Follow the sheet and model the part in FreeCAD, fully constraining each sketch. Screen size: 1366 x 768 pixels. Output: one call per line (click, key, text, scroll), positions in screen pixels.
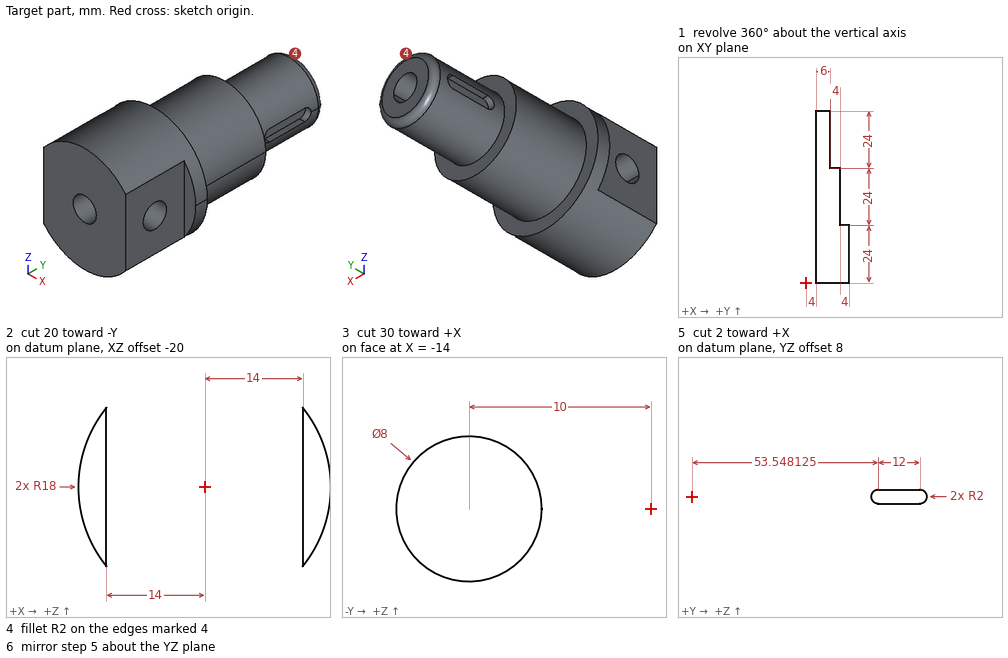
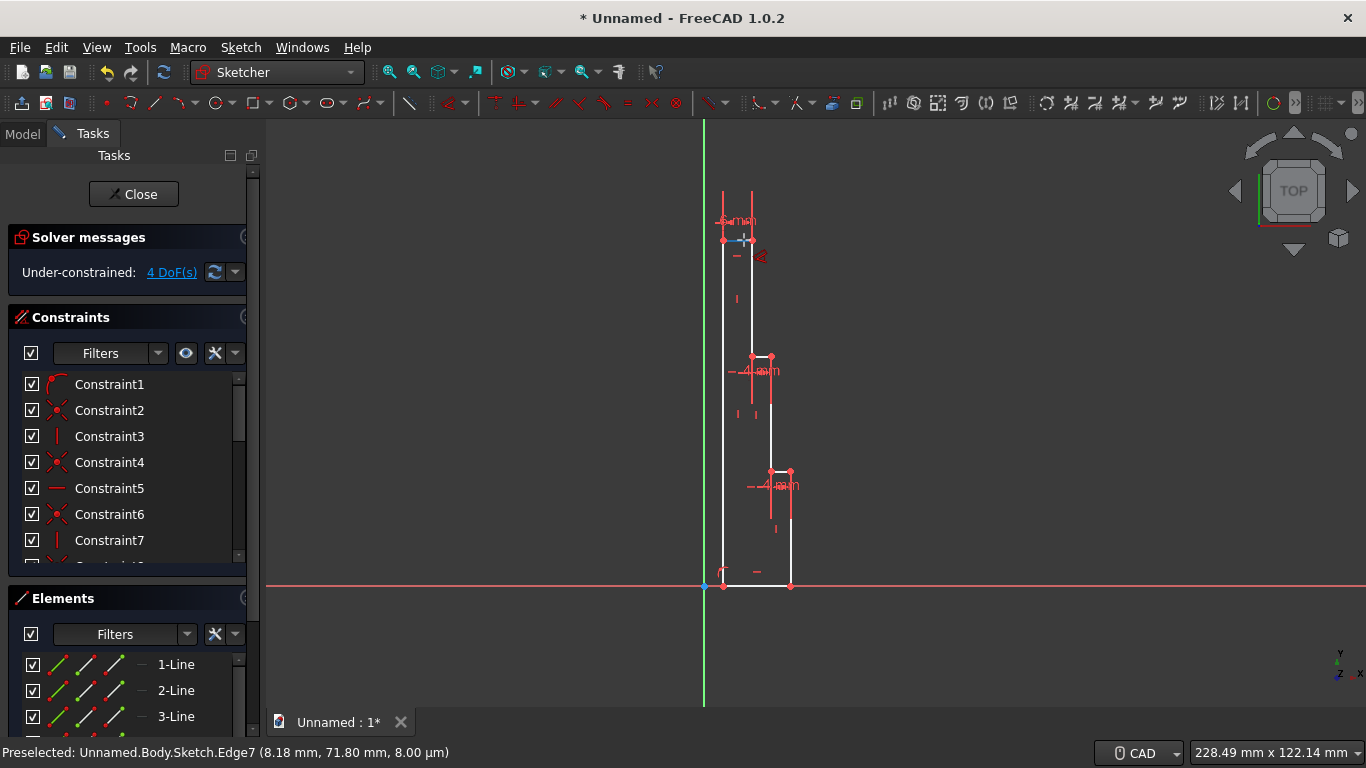
click(791, 552)
click(825, 529)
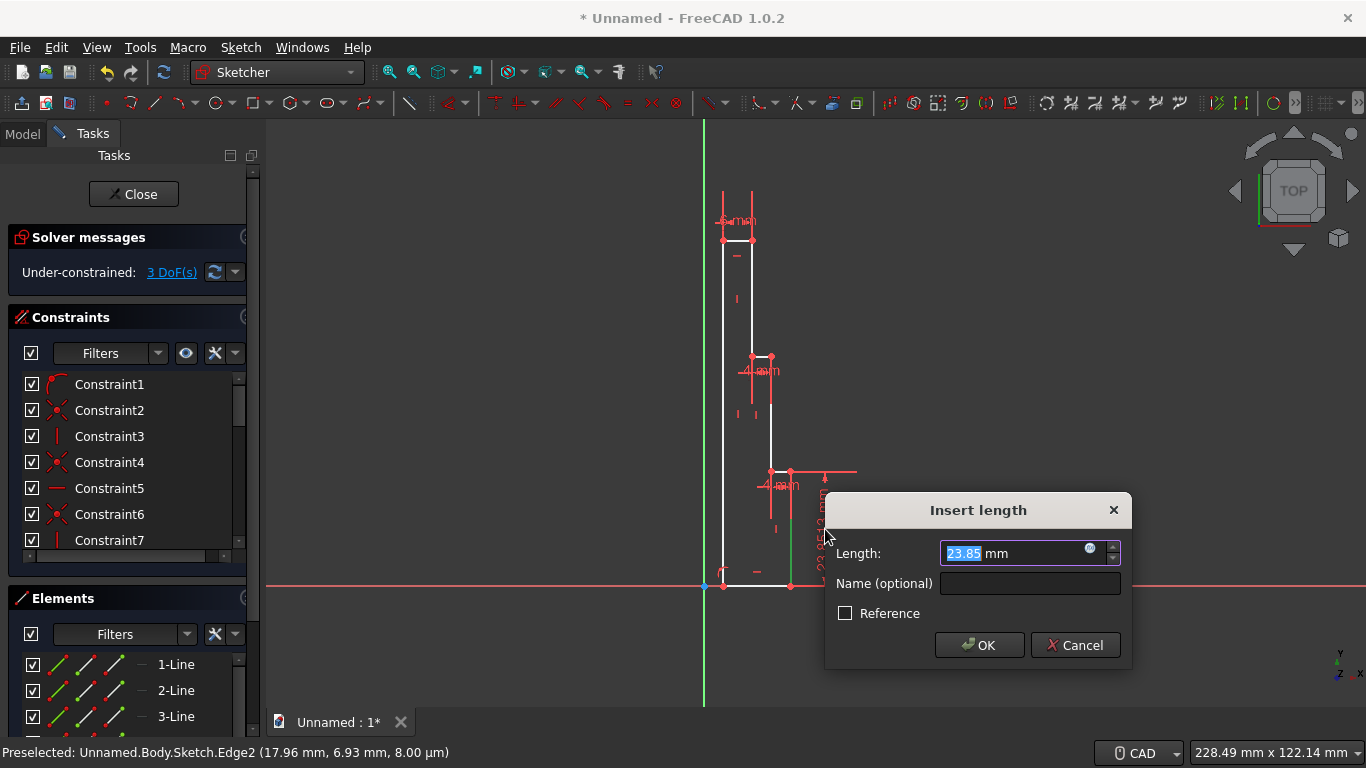
text(24)
key(Return)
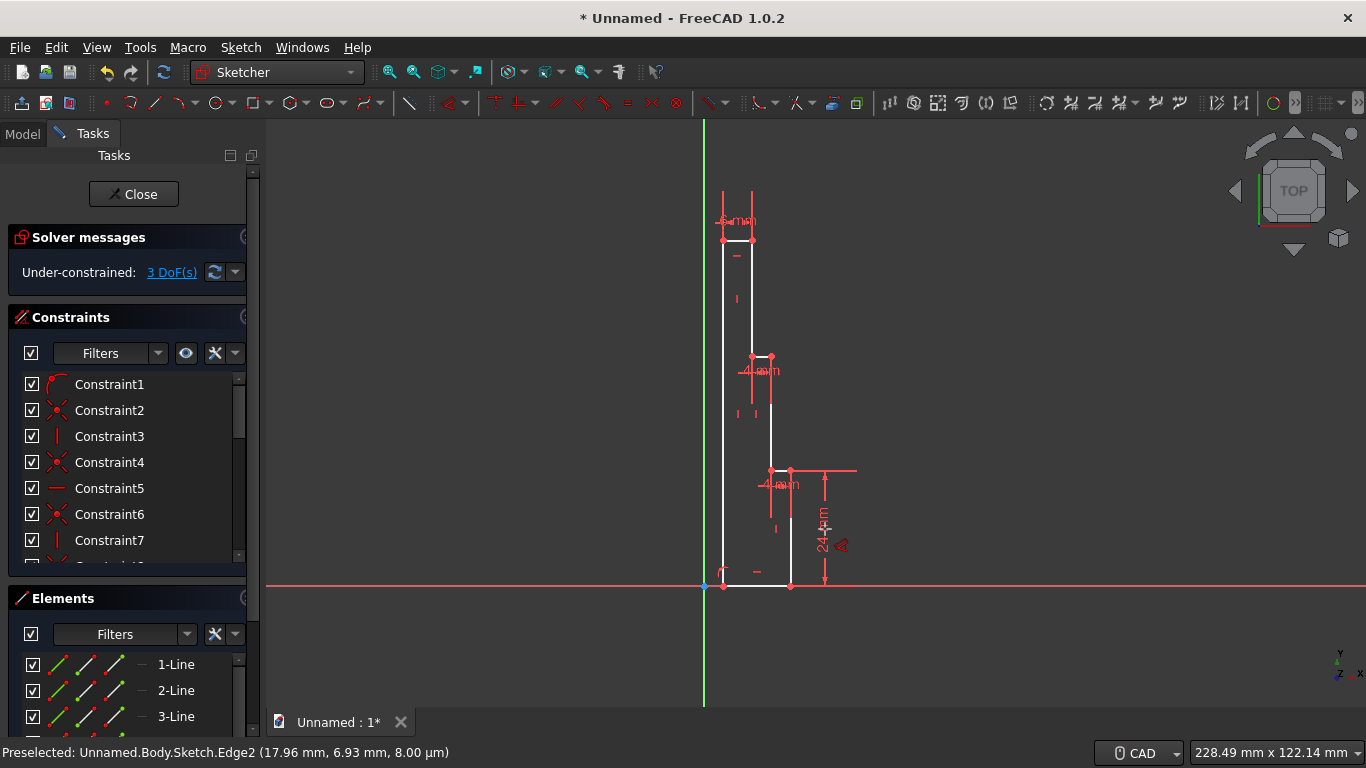
click(771, 437)
click(805, 414)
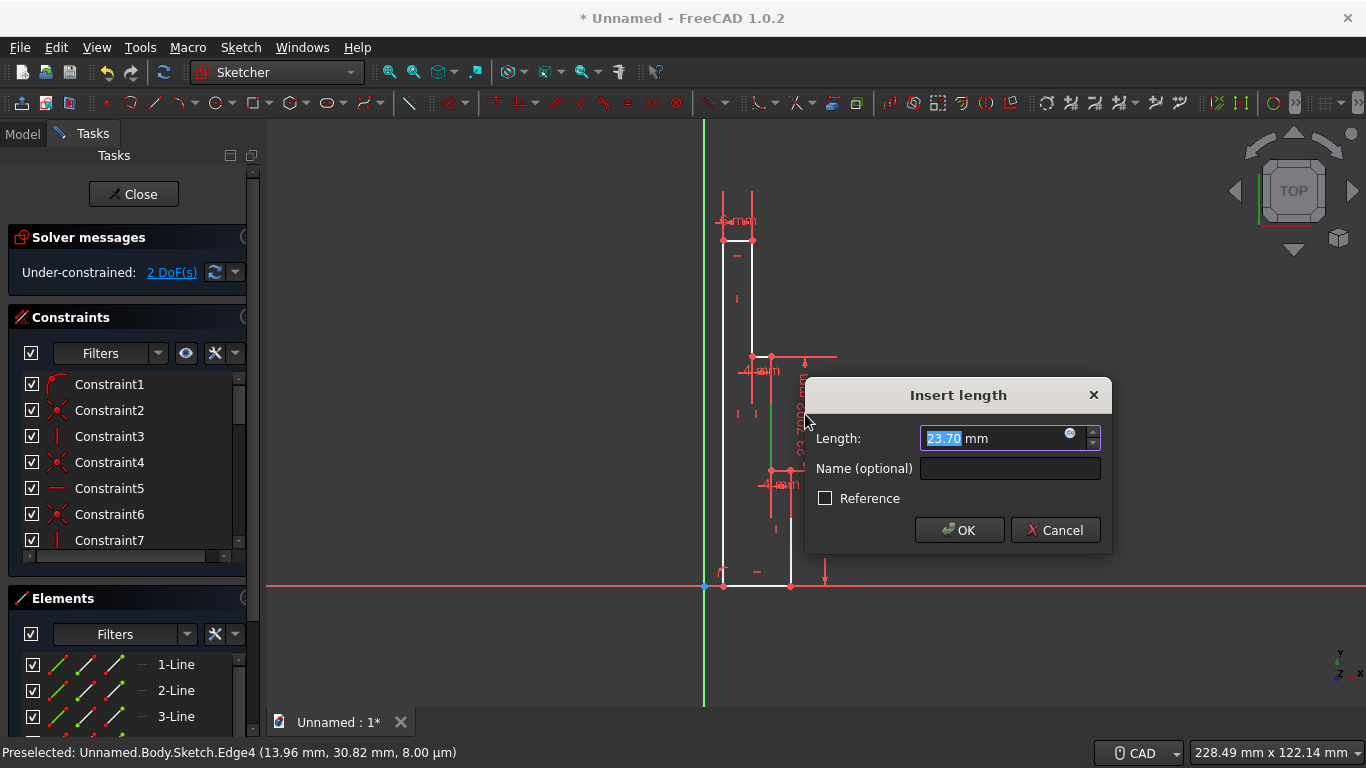
text(24)
key(Return)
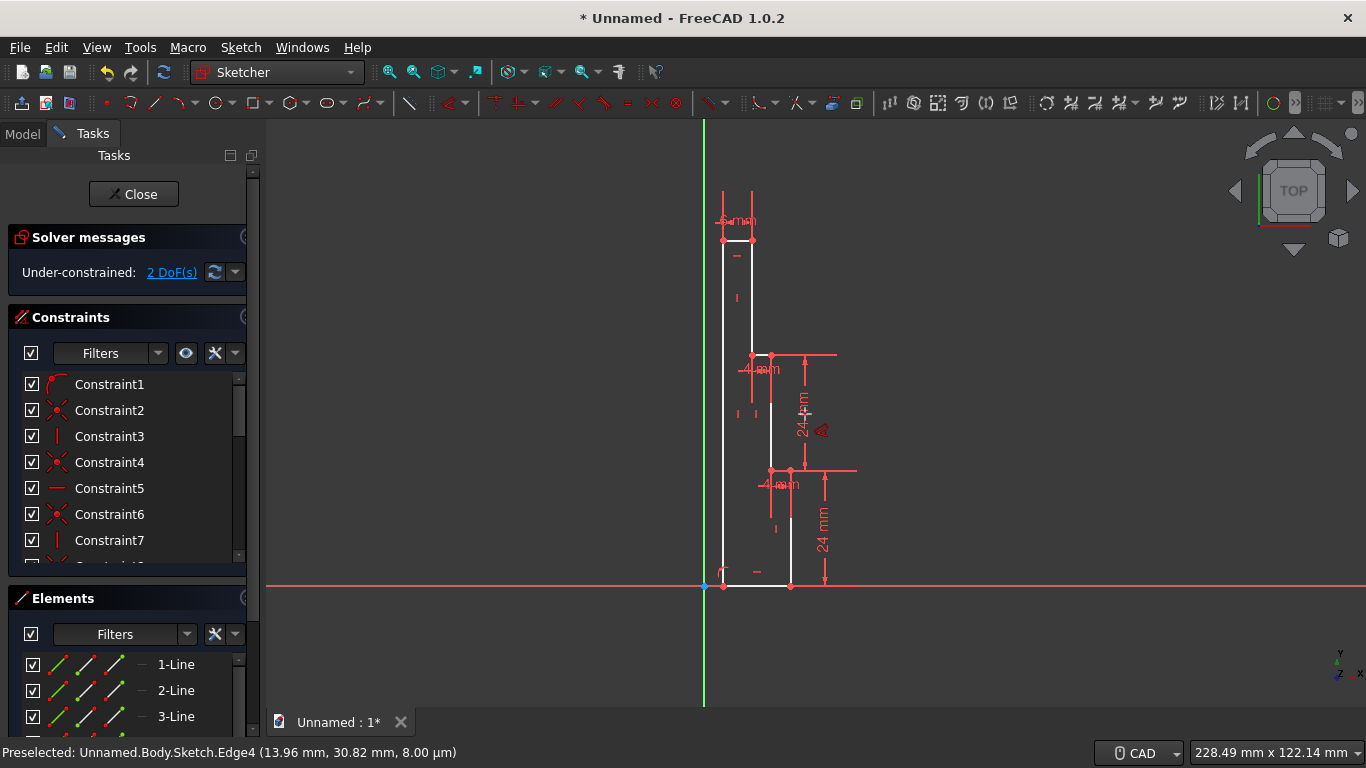
click(752, 321)
click(786, 298)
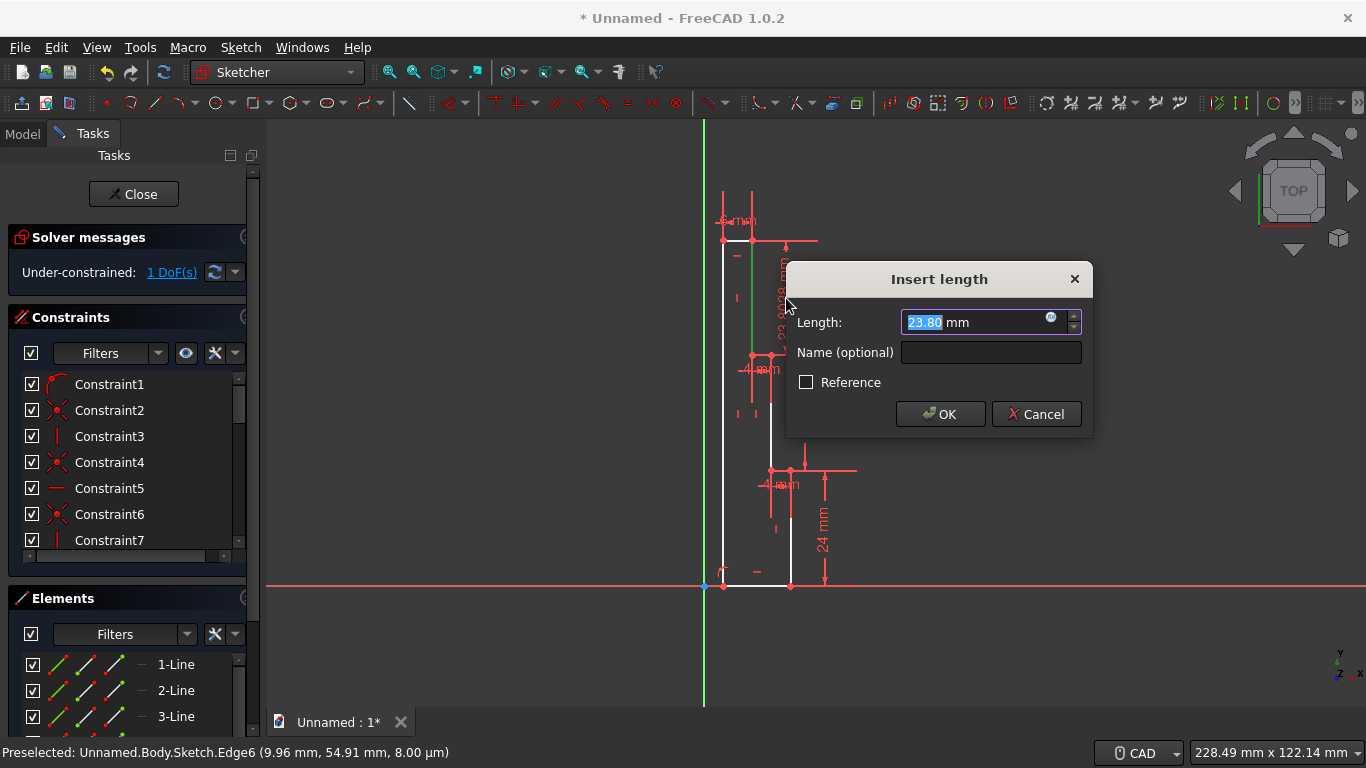
text(24)
key(Return)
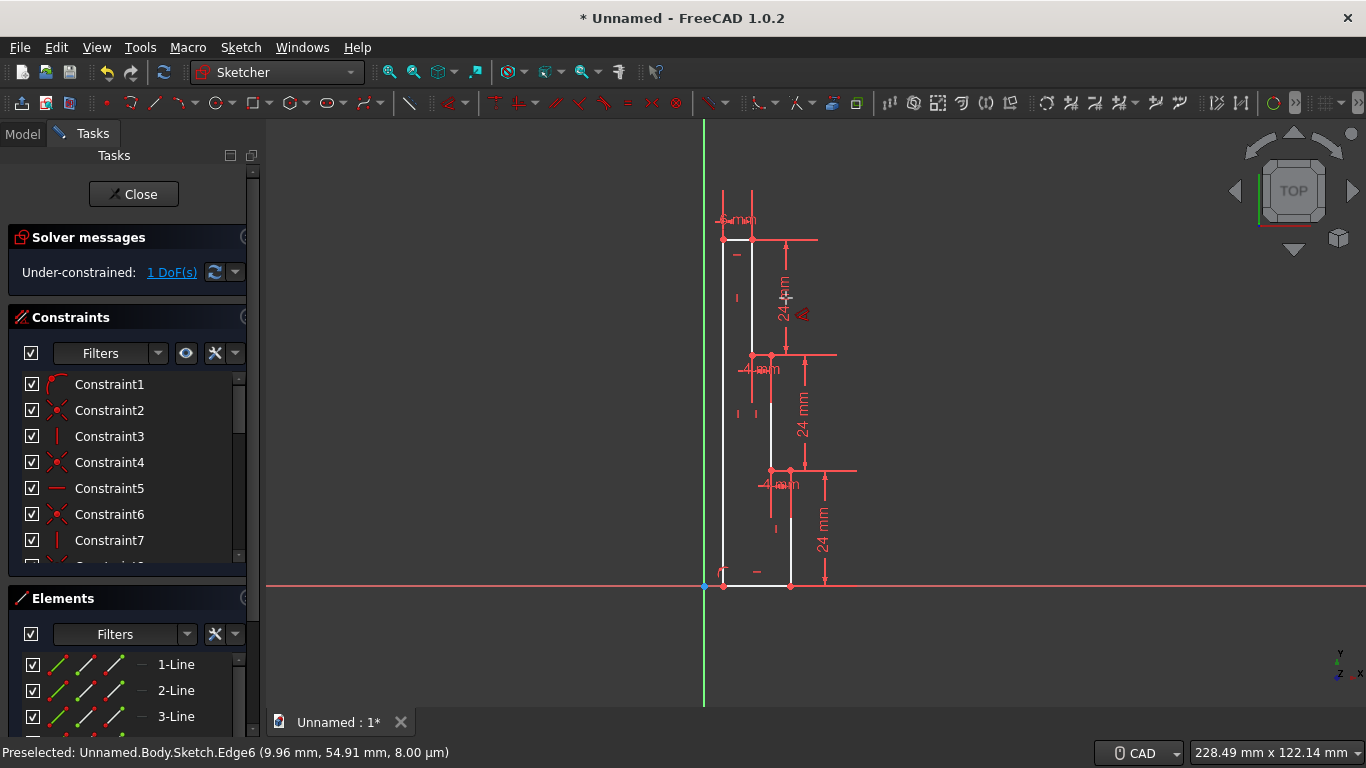
scroll(723, 586, up, 4)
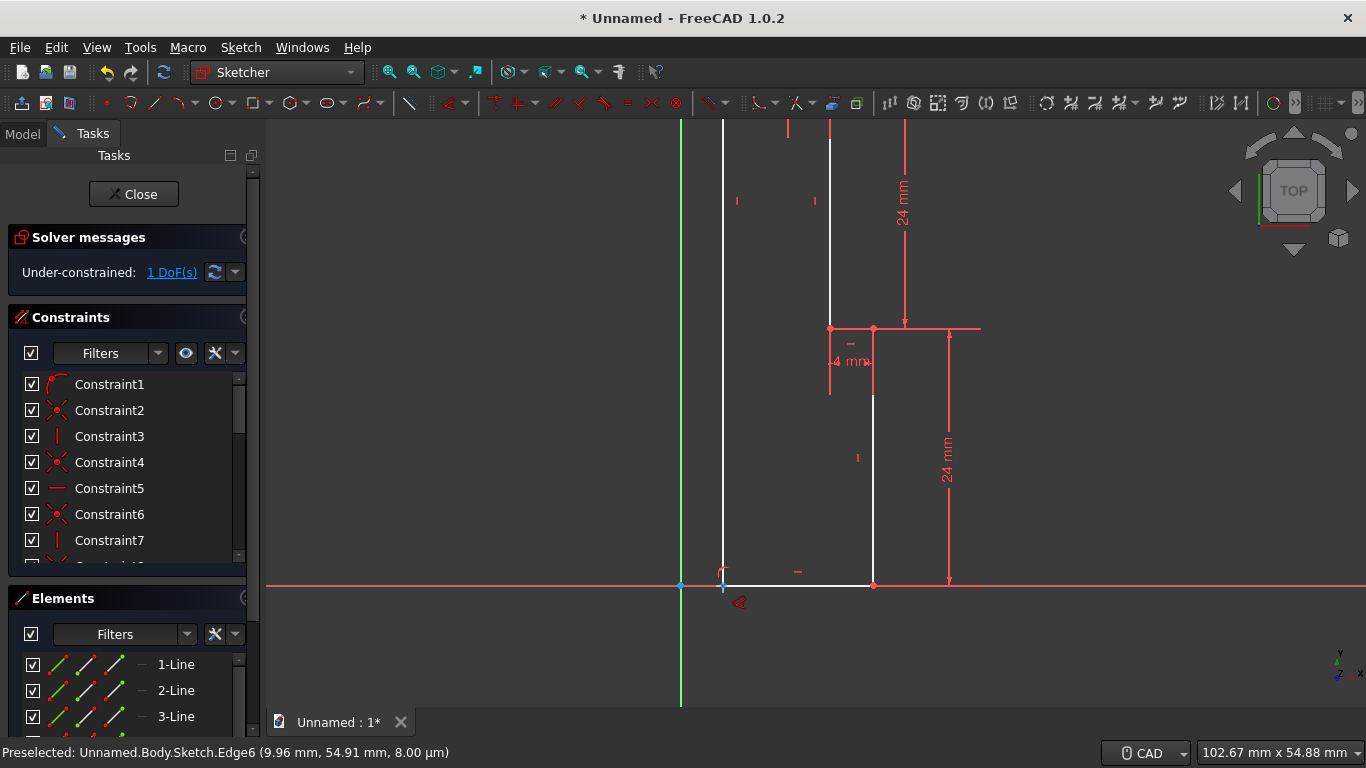
click(723, 586)
click(702, 620)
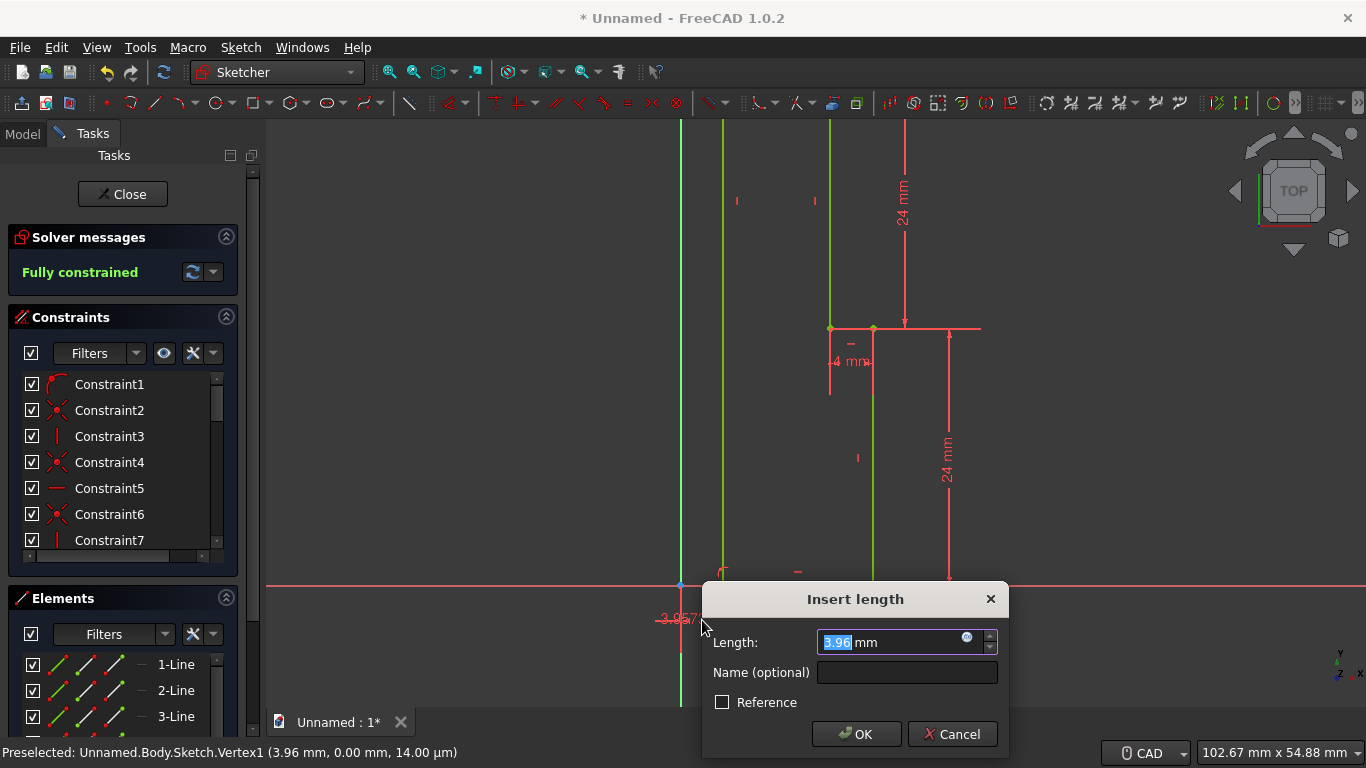
text(4)
key(Return)
key(Escape)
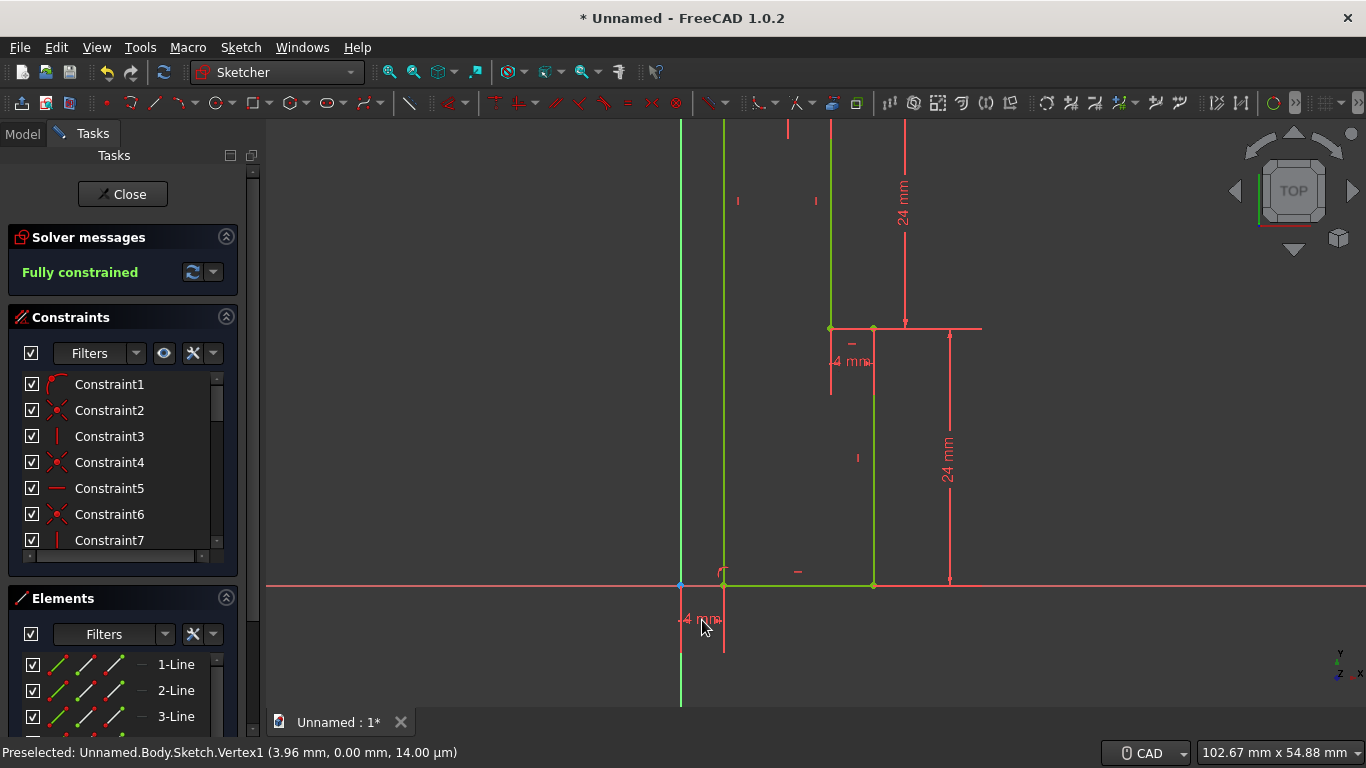
click(123, 194)